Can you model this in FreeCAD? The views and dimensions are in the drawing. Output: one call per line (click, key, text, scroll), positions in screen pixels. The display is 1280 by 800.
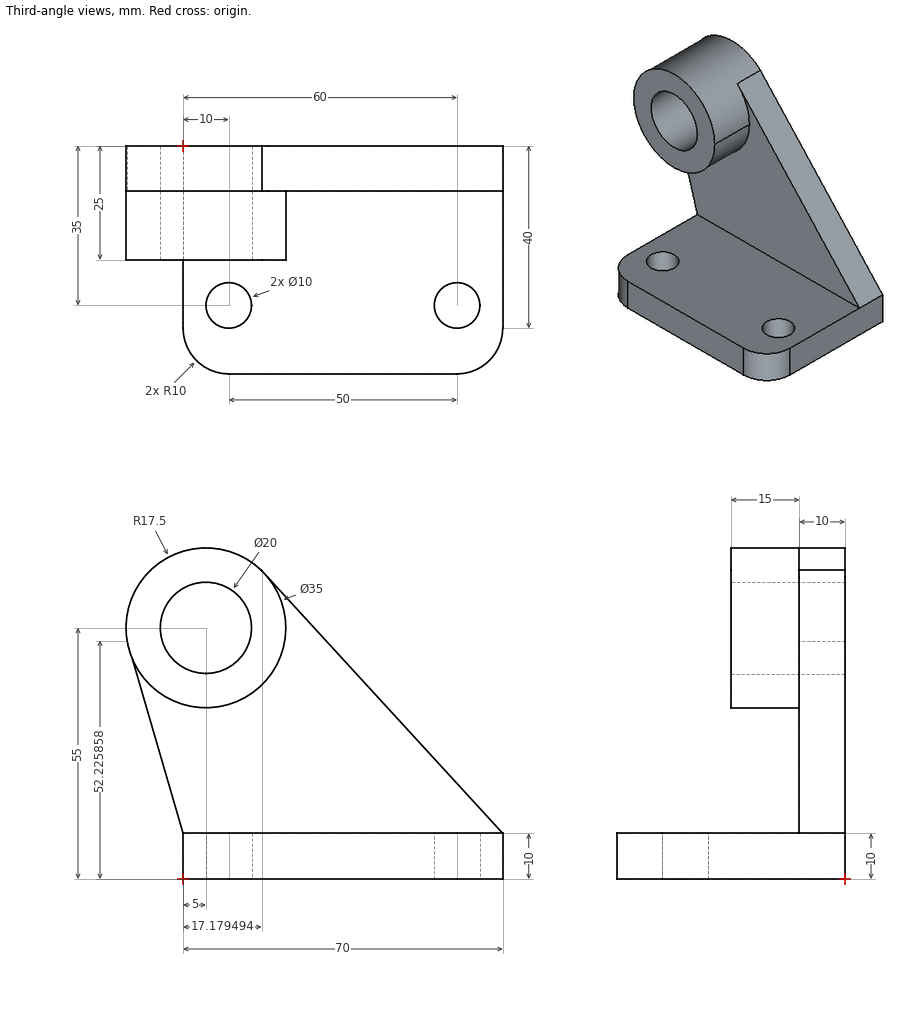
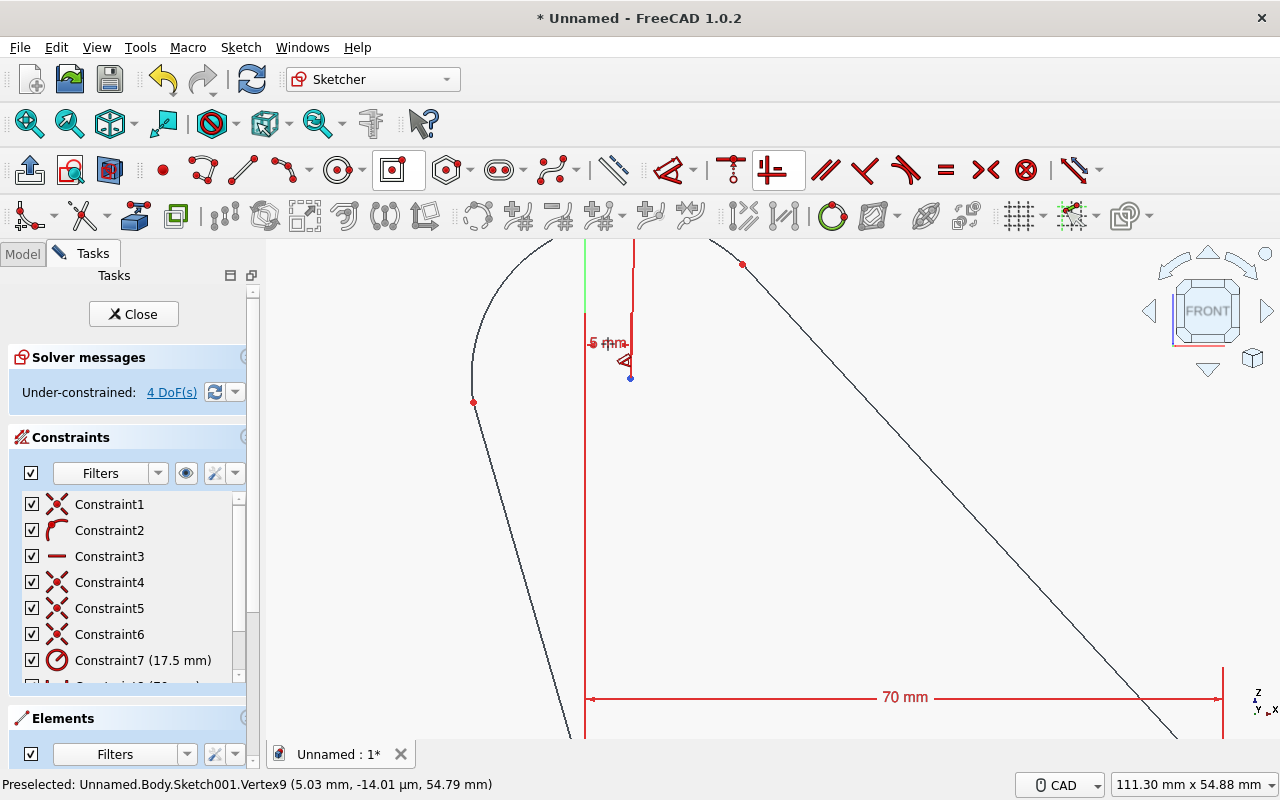
scroll(587, 434, down, 4)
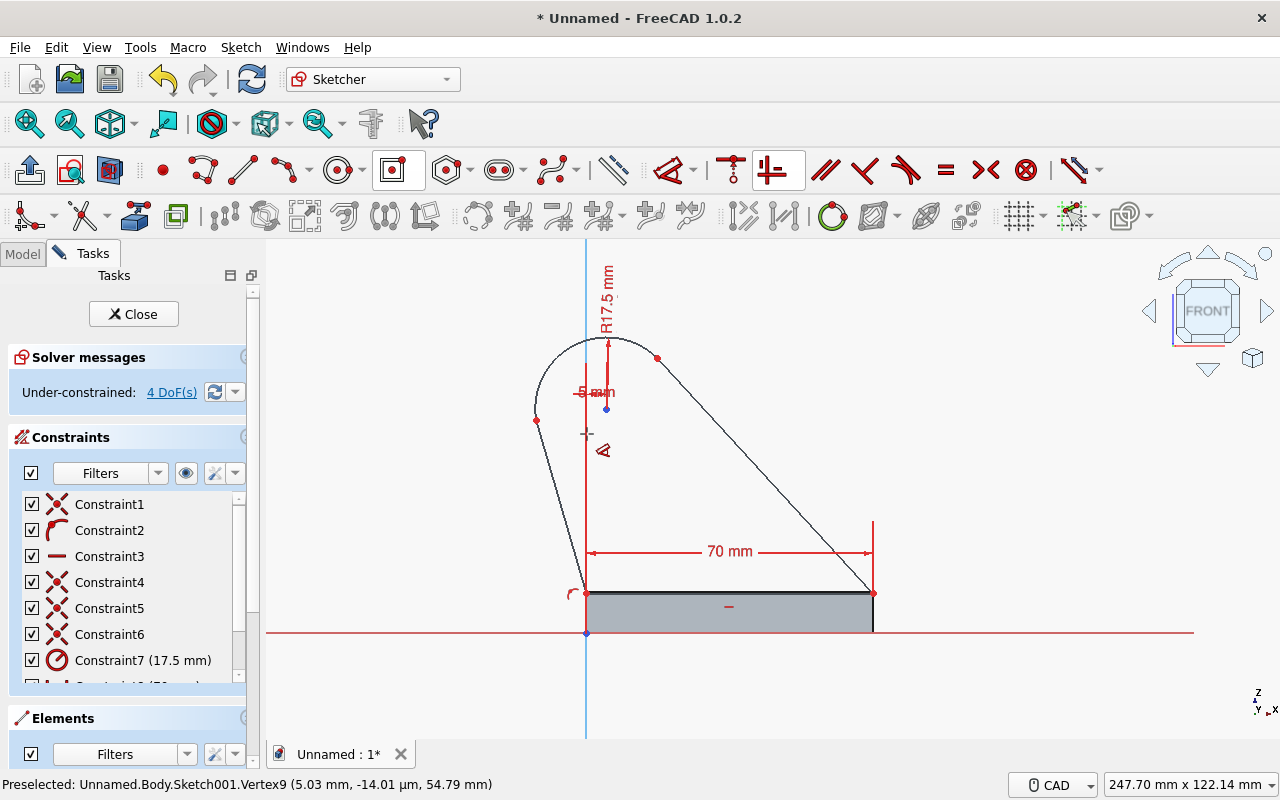
click(873, 594)
click(907, 614)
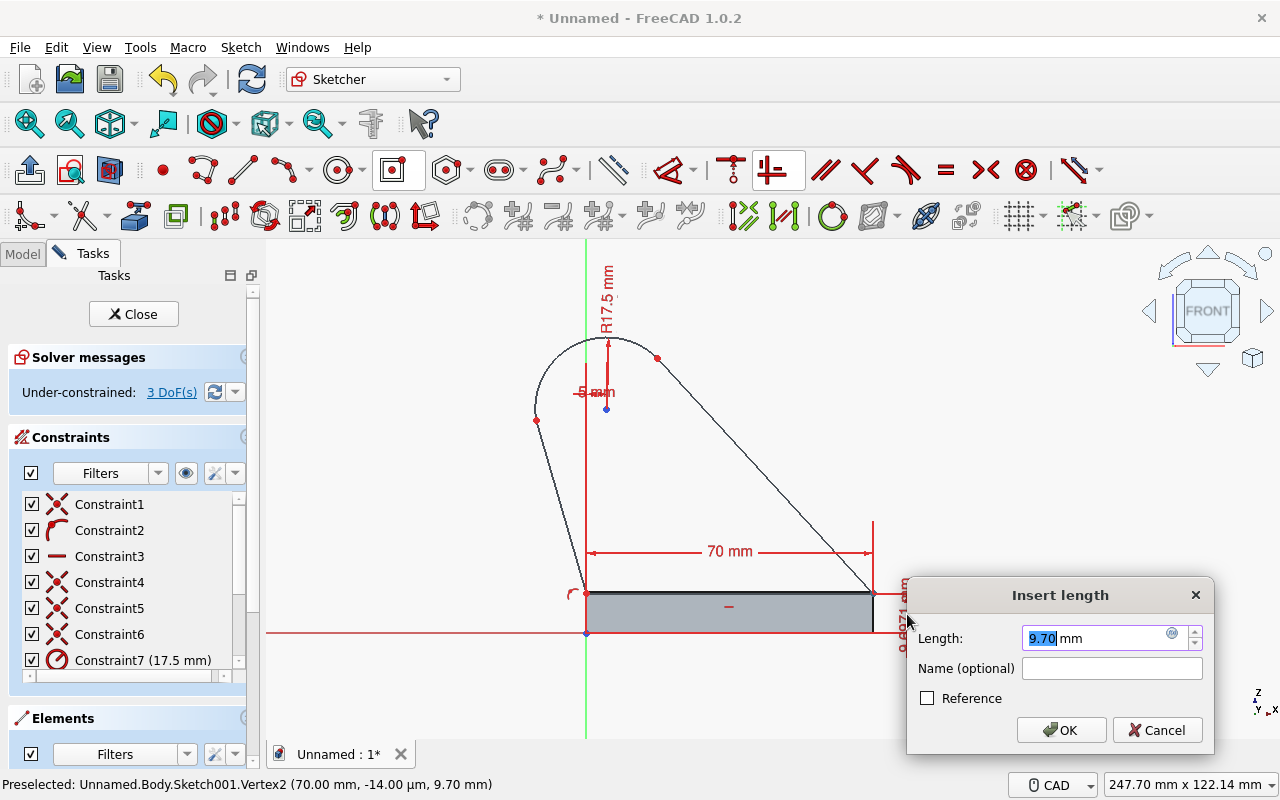
text(10)
key(Return)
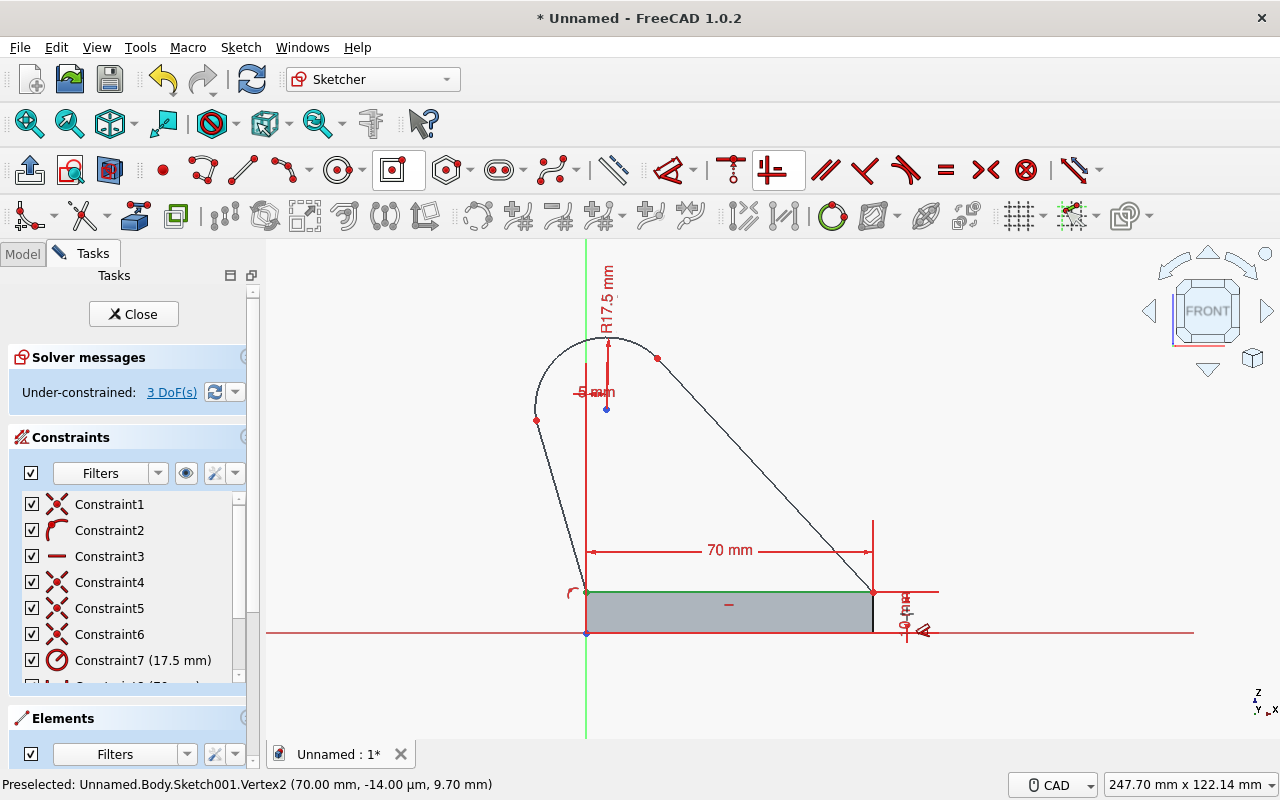
click(607, 409)
click(552, 573)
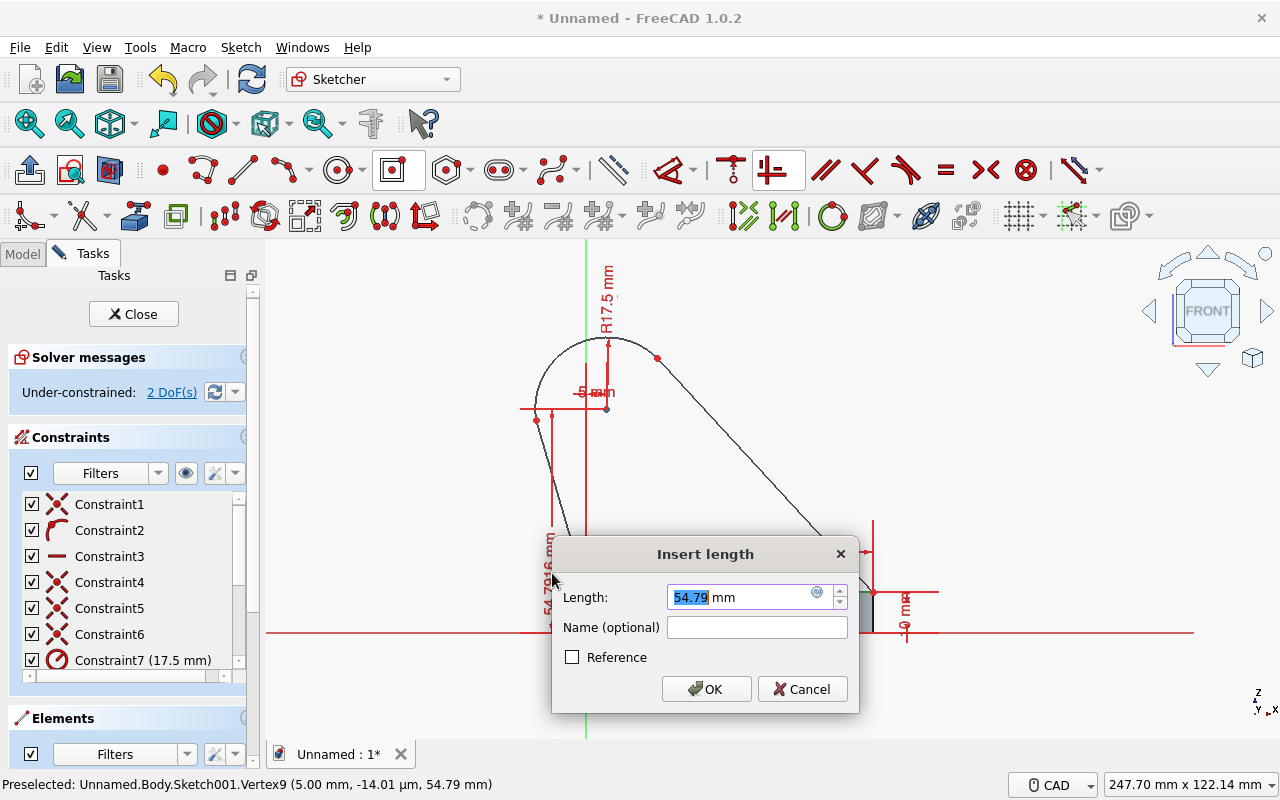
text(55)
key(Return)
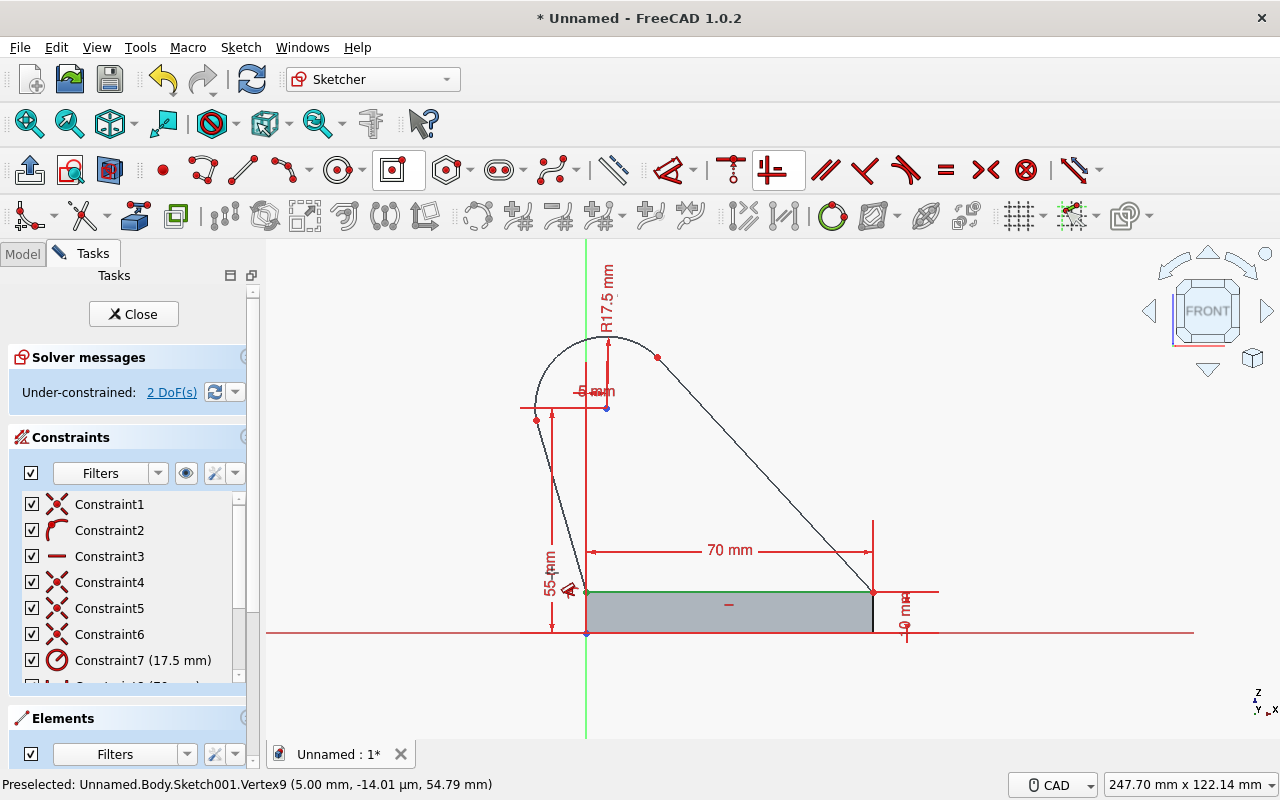
click(657, 357)
click(622, 667)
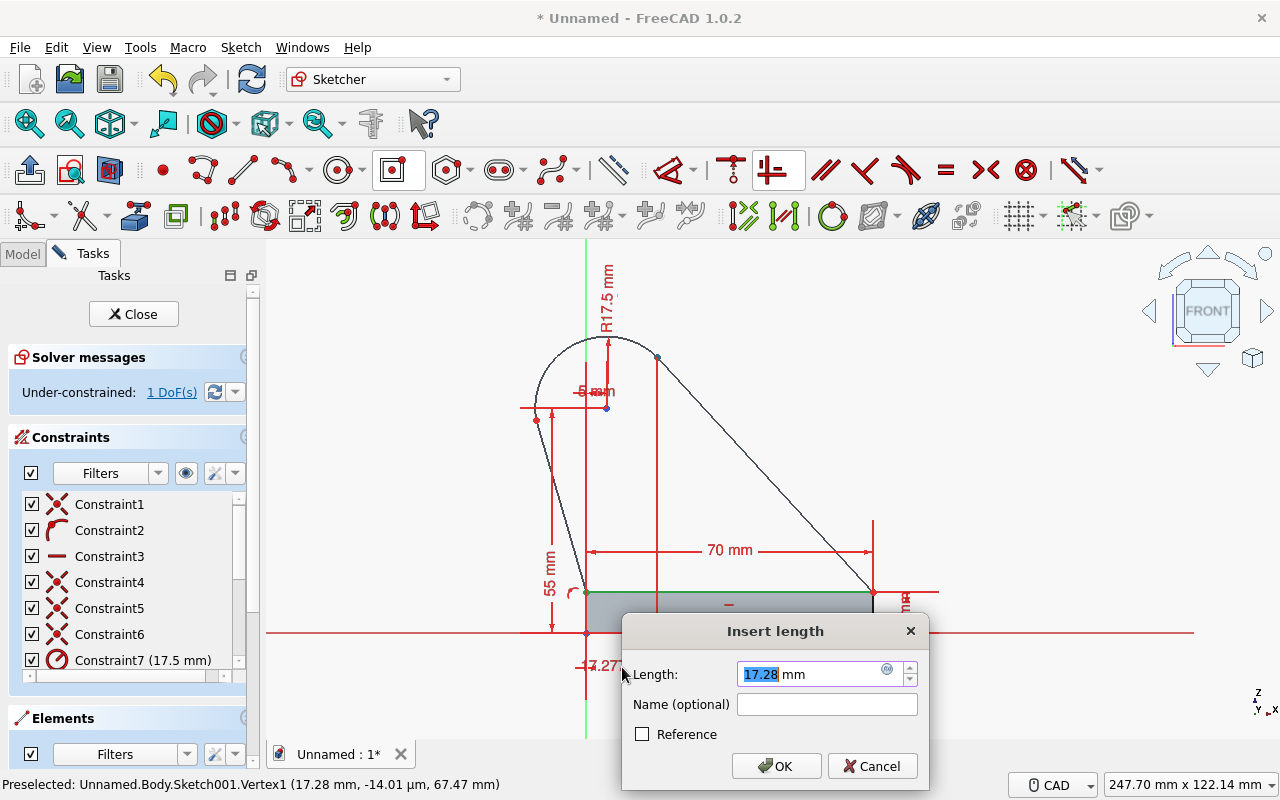
text(17.179494)
key(Return)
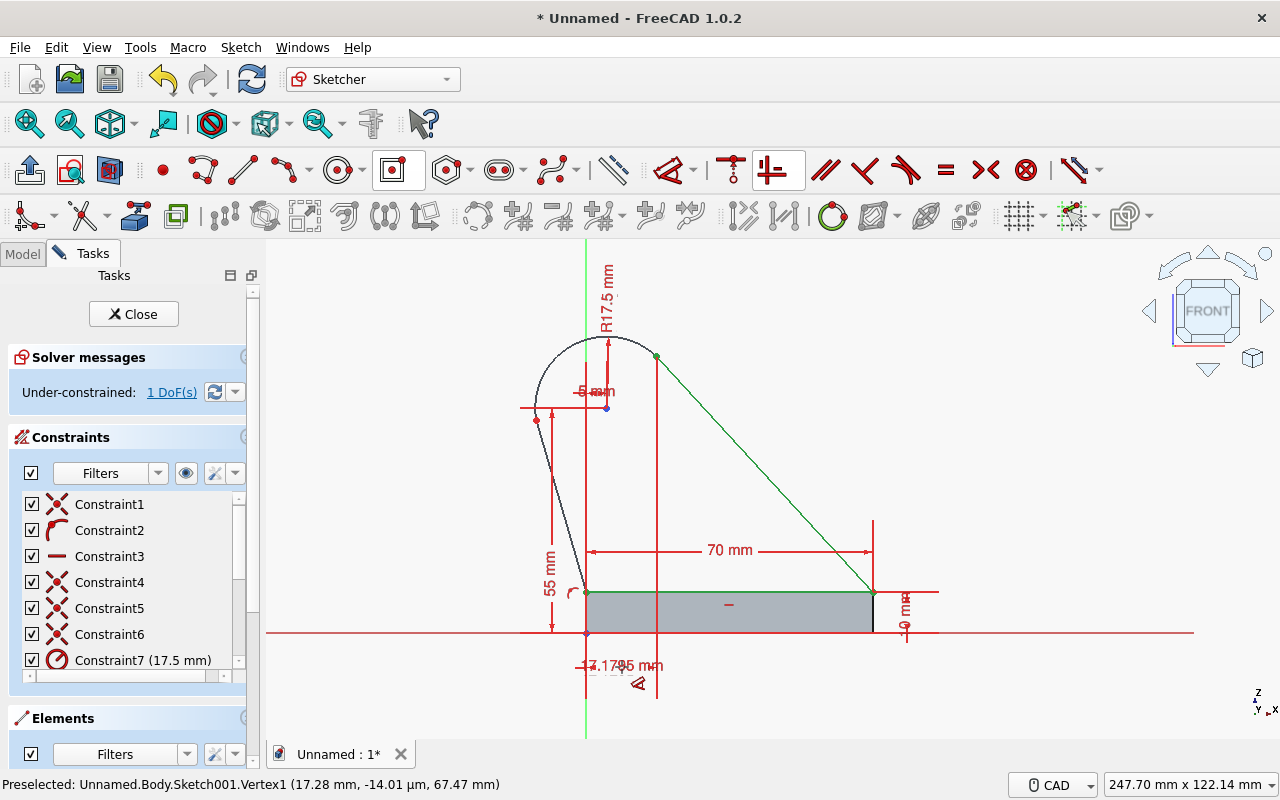
click(536, 420)
click(502, 527)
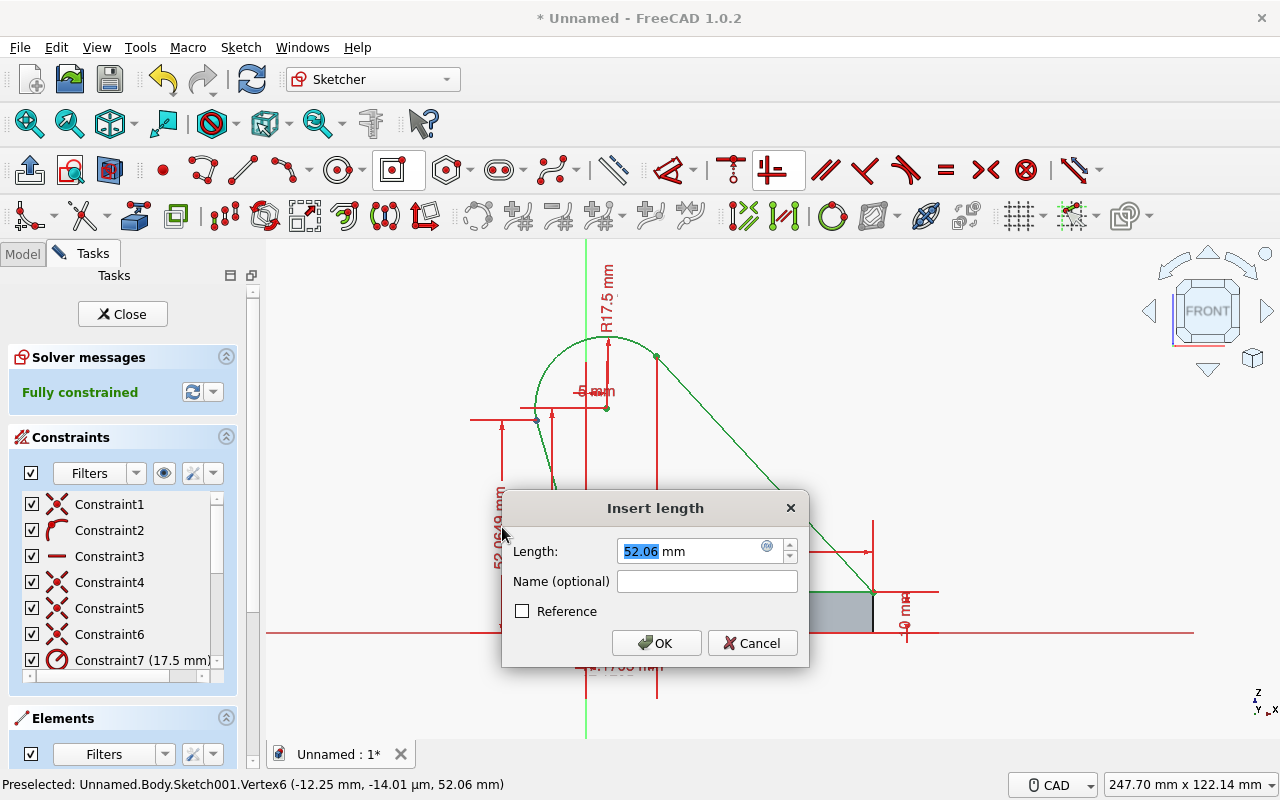
text(52.225858)
key(Return)
key(Escape)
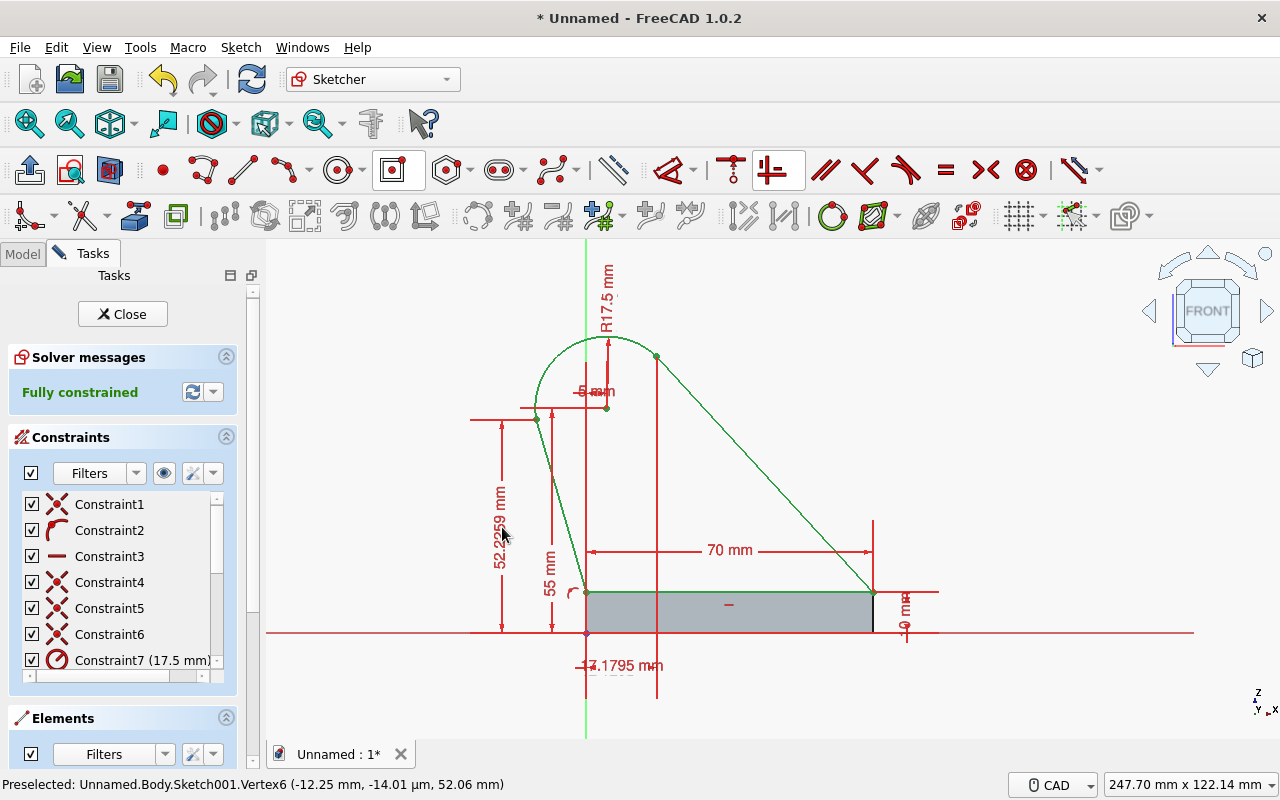
click(123, 314)